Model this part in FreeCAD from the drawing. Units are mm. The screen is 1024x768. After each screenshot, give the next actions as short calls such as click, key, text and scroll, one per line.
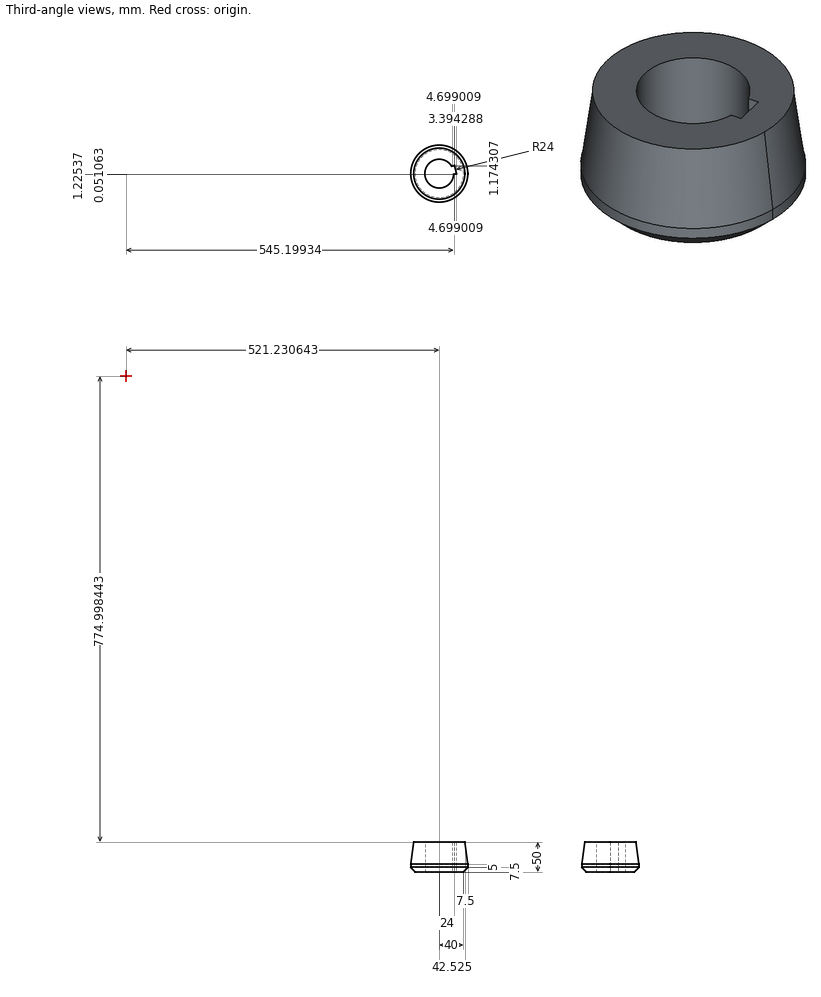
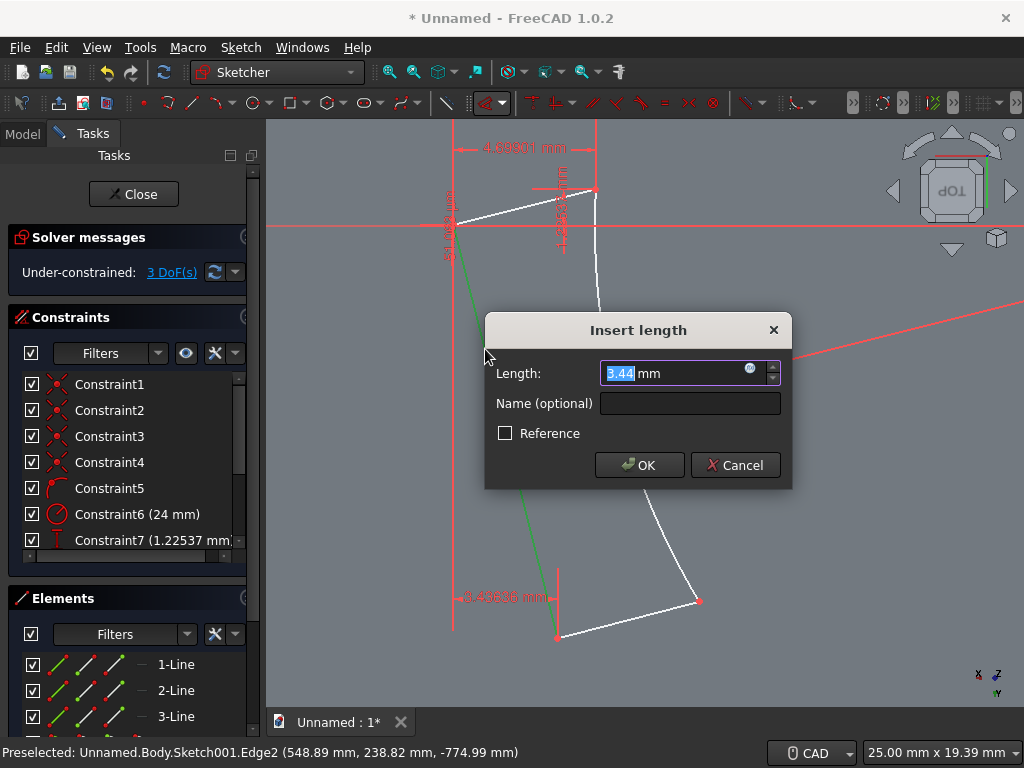
text(3.394288)
key(Return)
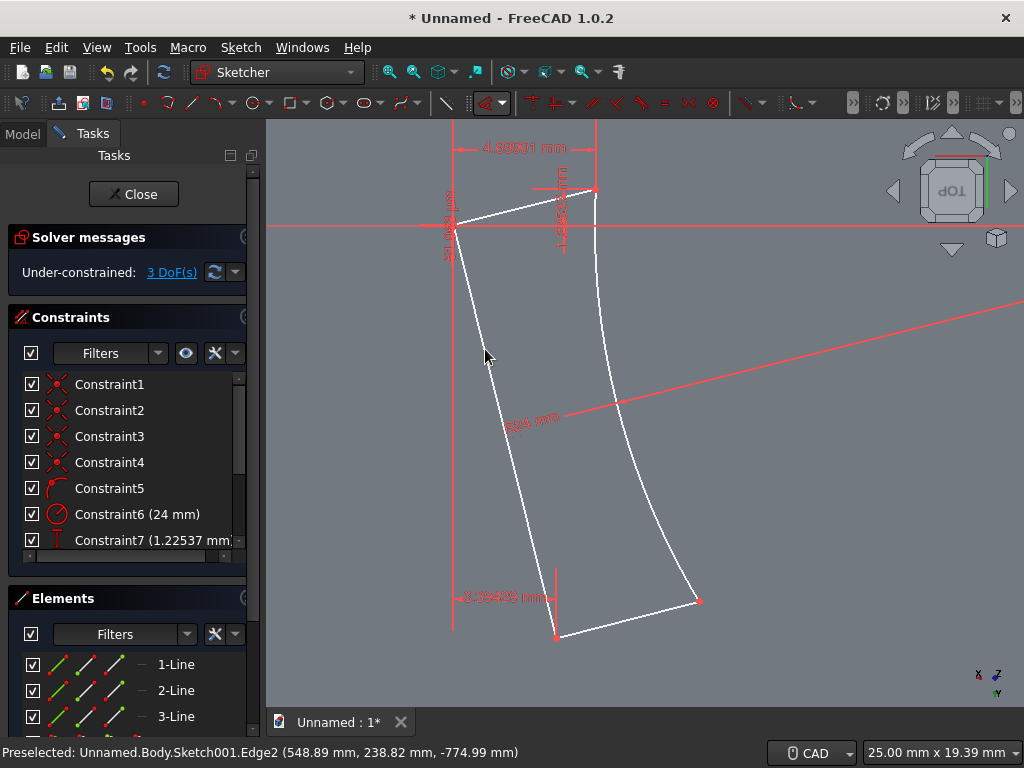
click(599, 627)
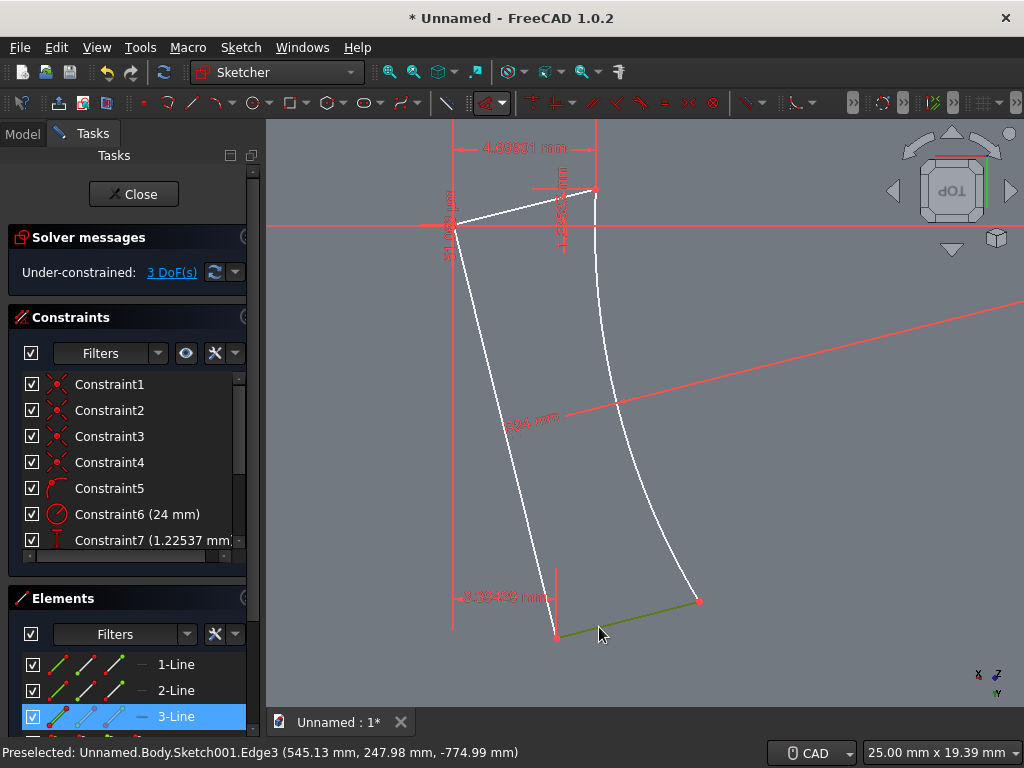
click(504, 104)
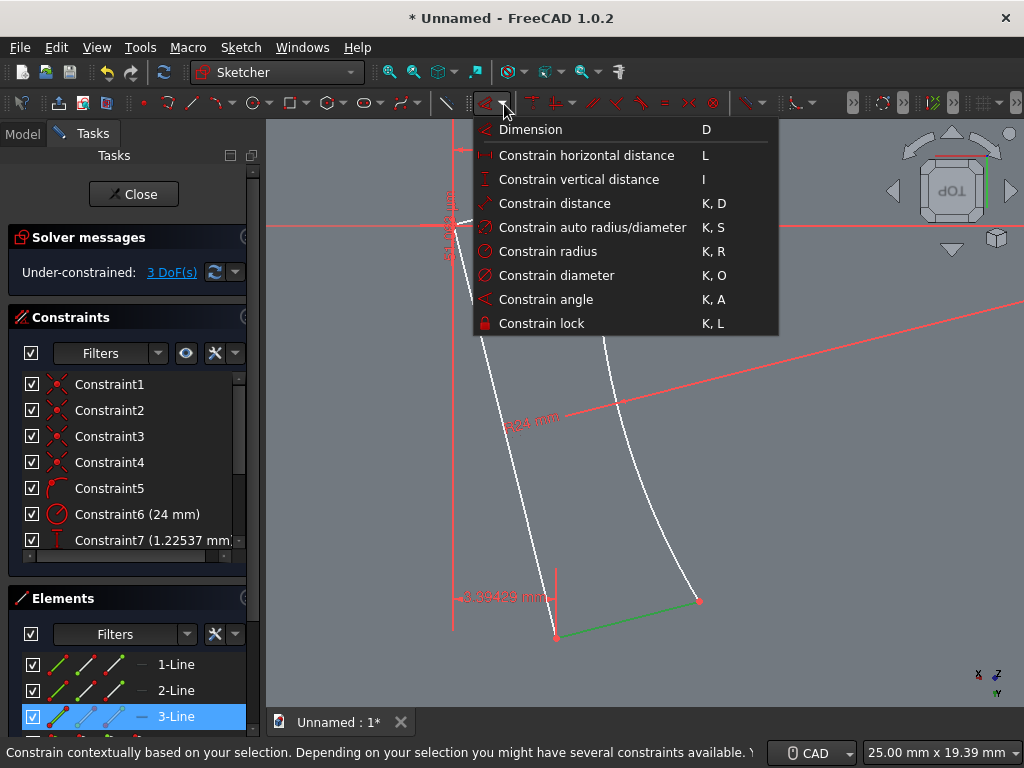
click(626, 155)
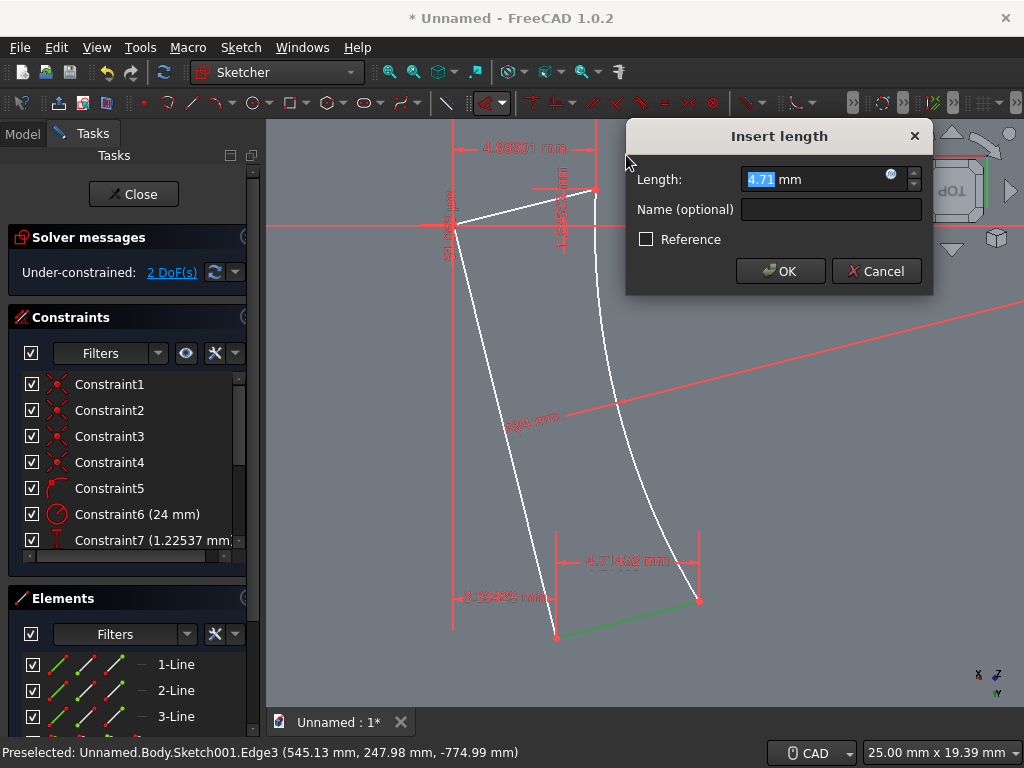
text(4.699009)
key(Return)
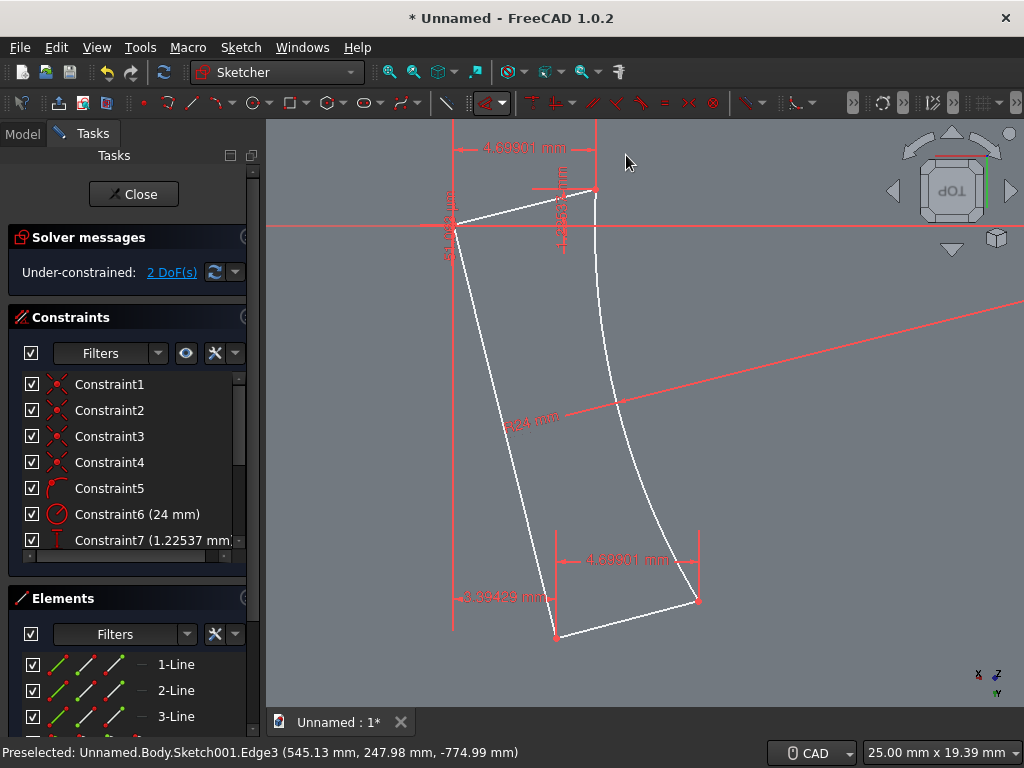
click(599, 627)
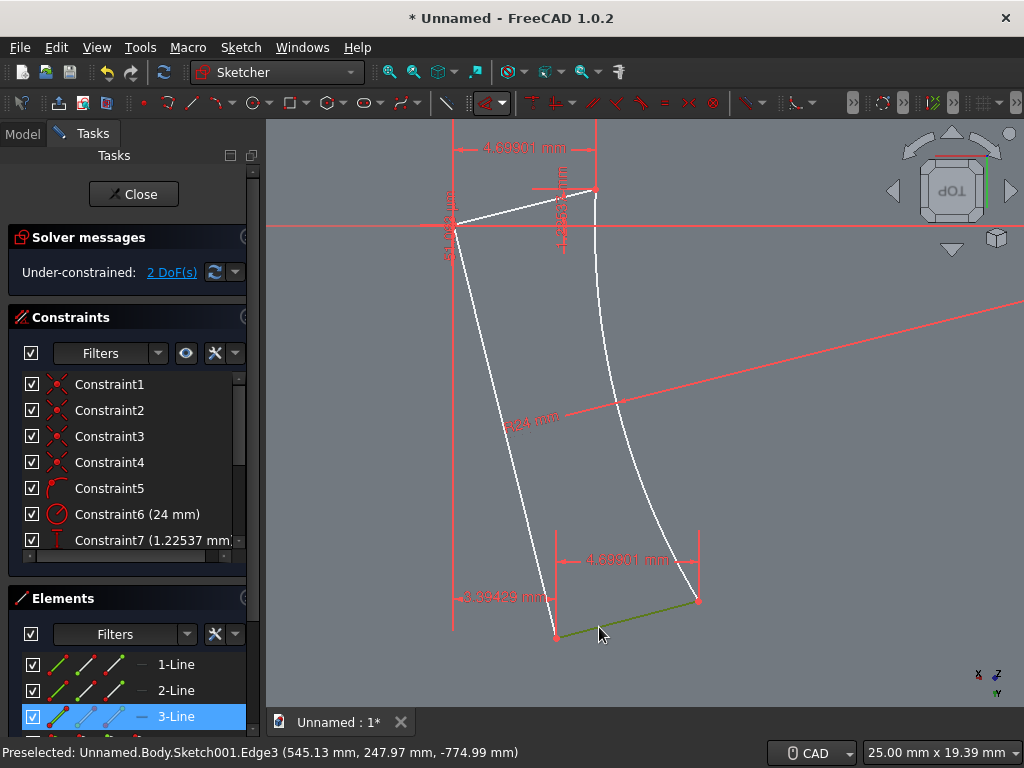
key(i)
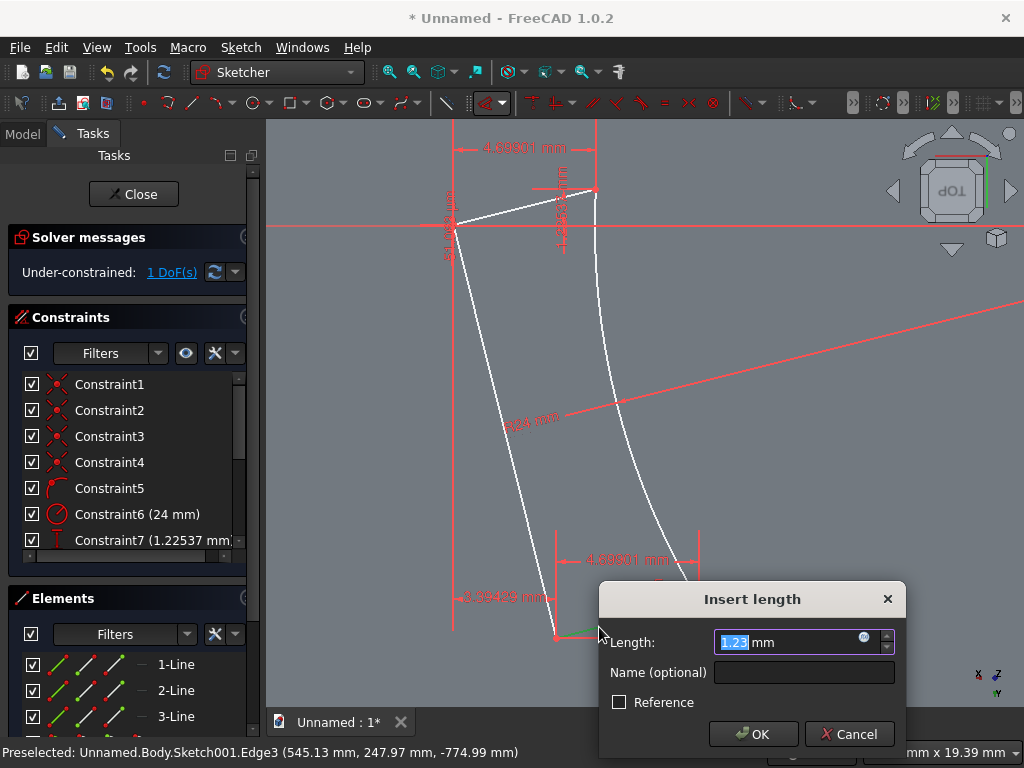
text(1.174307)
key(Return)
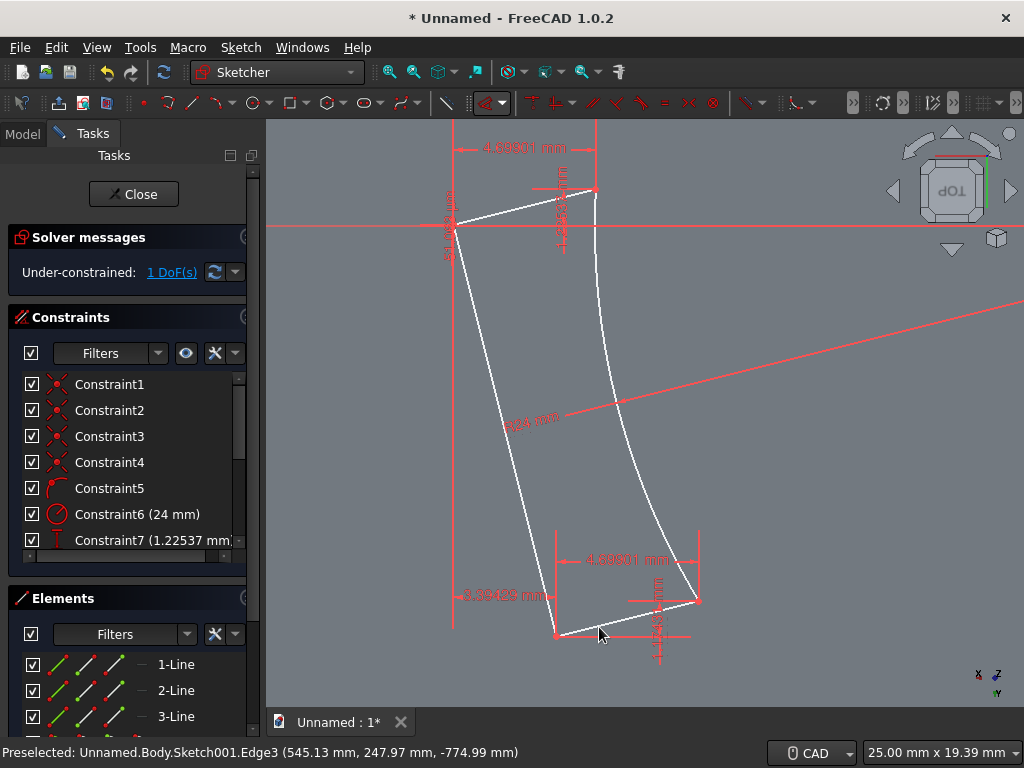
click(596, 189)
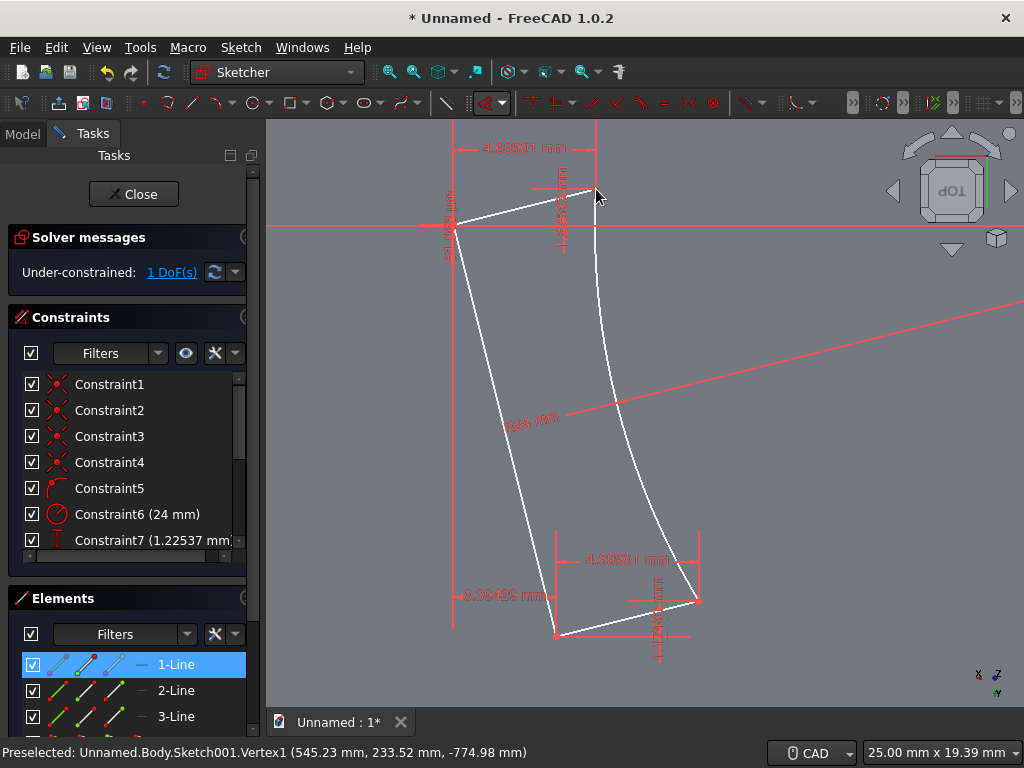
key(l)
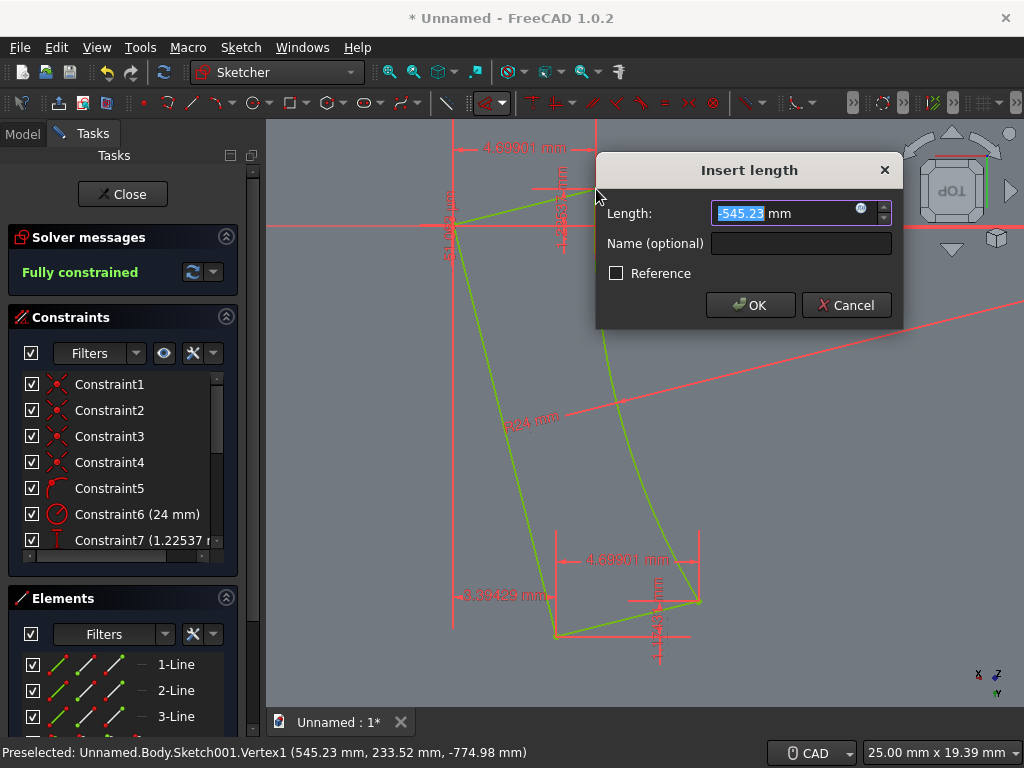
text(-545.19934)
key(Return)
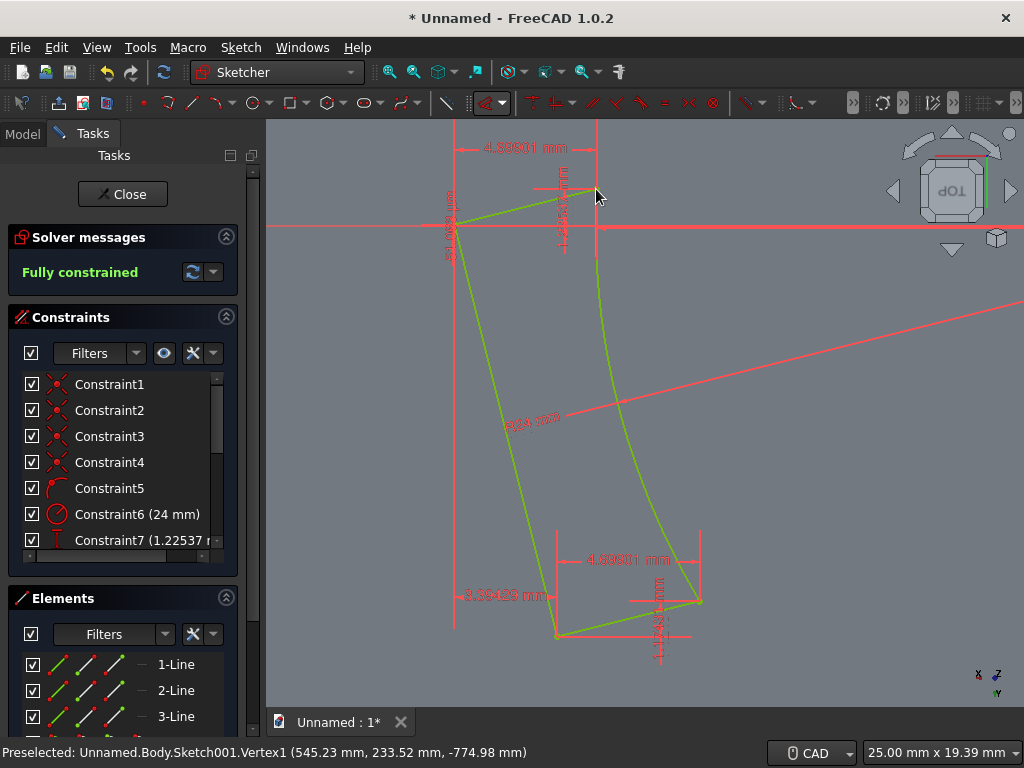
click(123, 194)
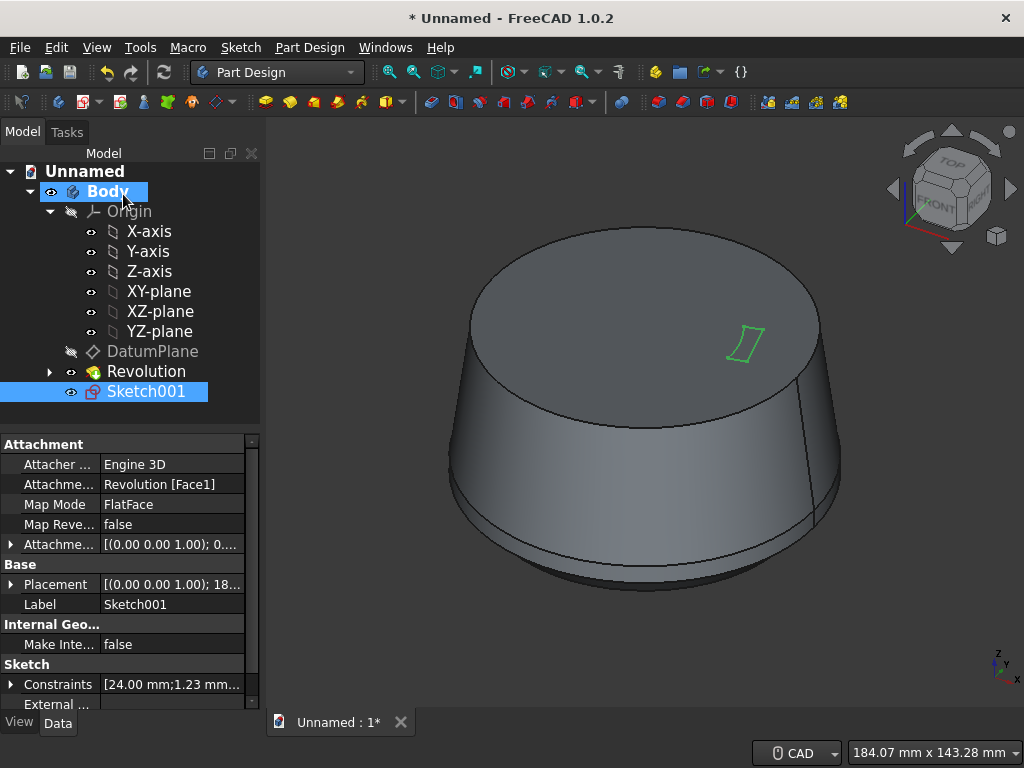
click(432, 102)